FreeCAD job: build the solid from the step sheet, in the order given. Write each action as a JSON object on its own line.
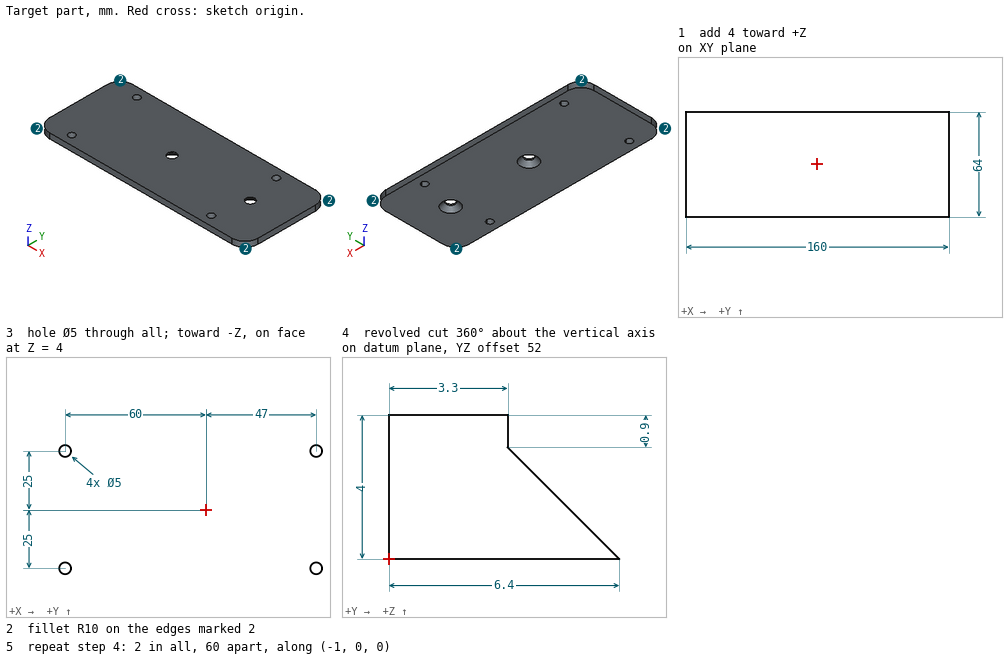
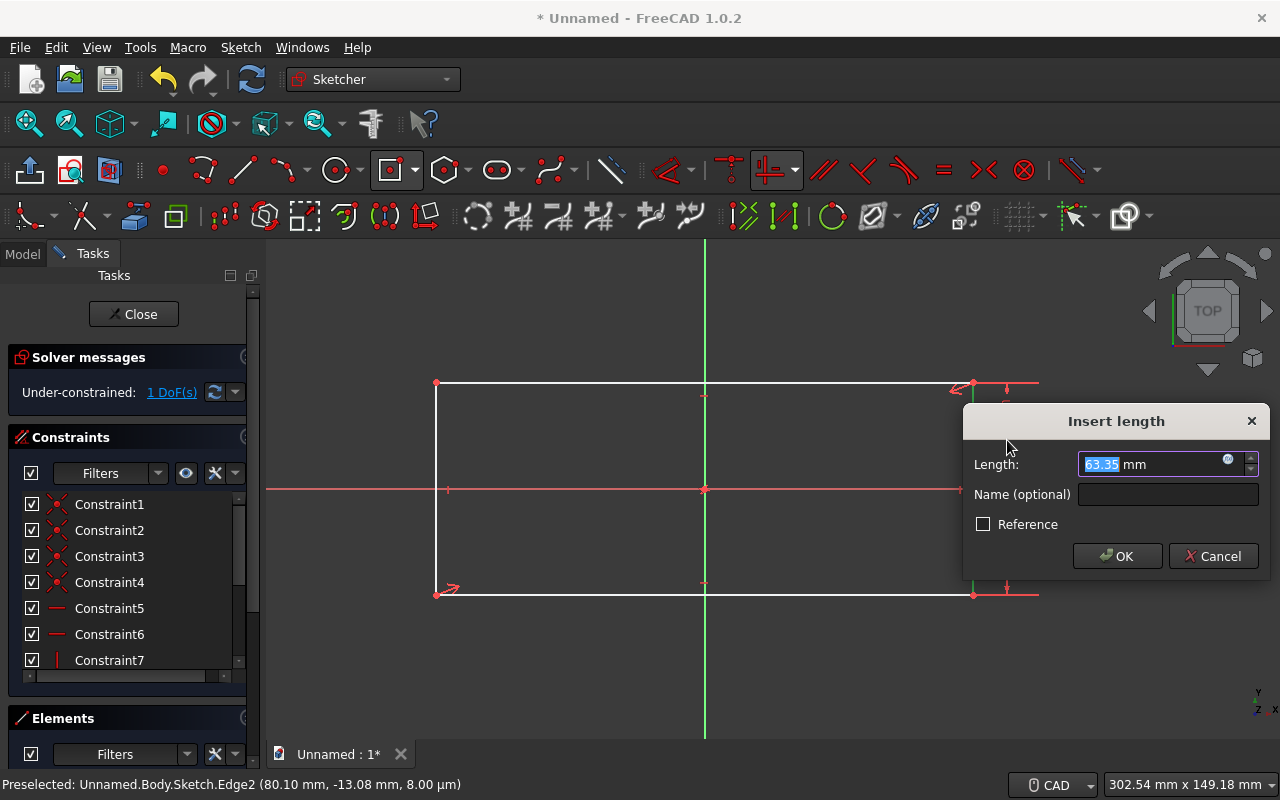
{"action": "type", "text": "64"}
{"action": "key", "text": "Return"}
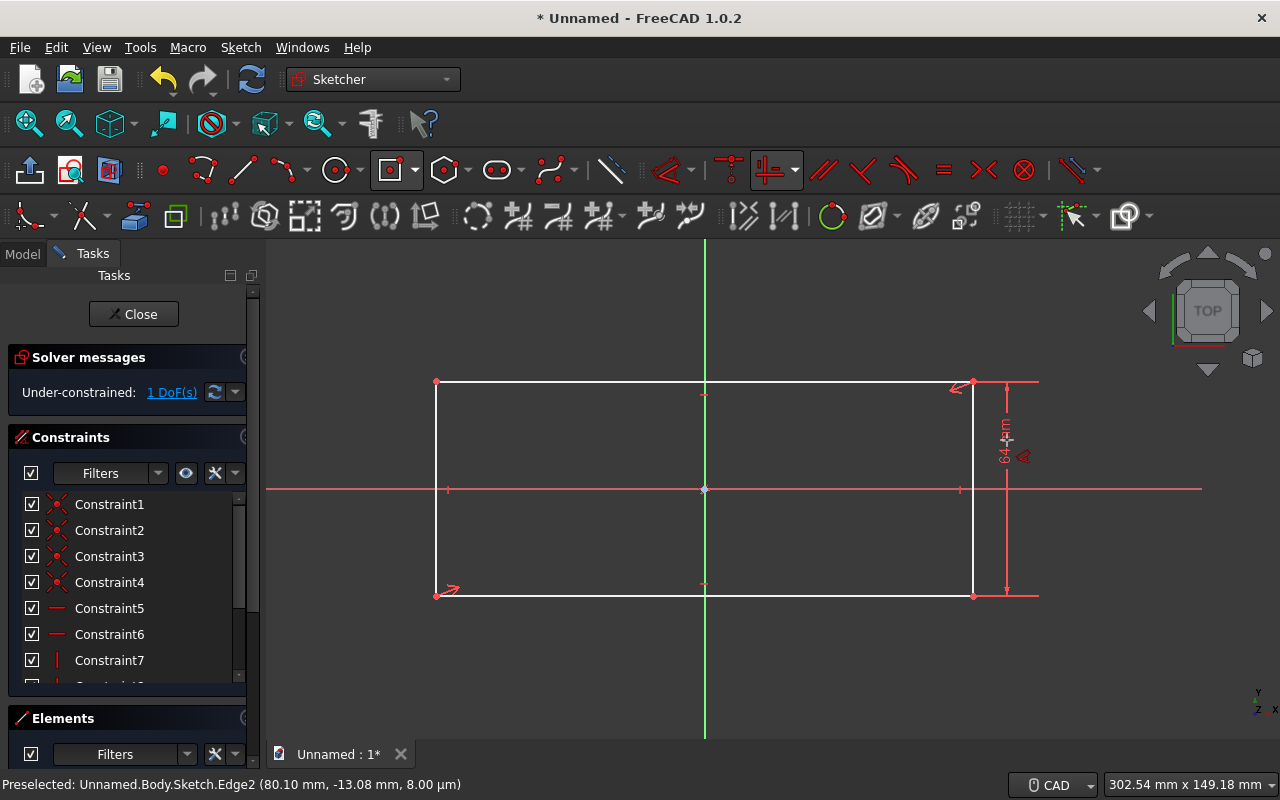
{"action": "left_click", "coordinate": [597, 596]}
{"action": "left_click", "coordinate": [581, 630]}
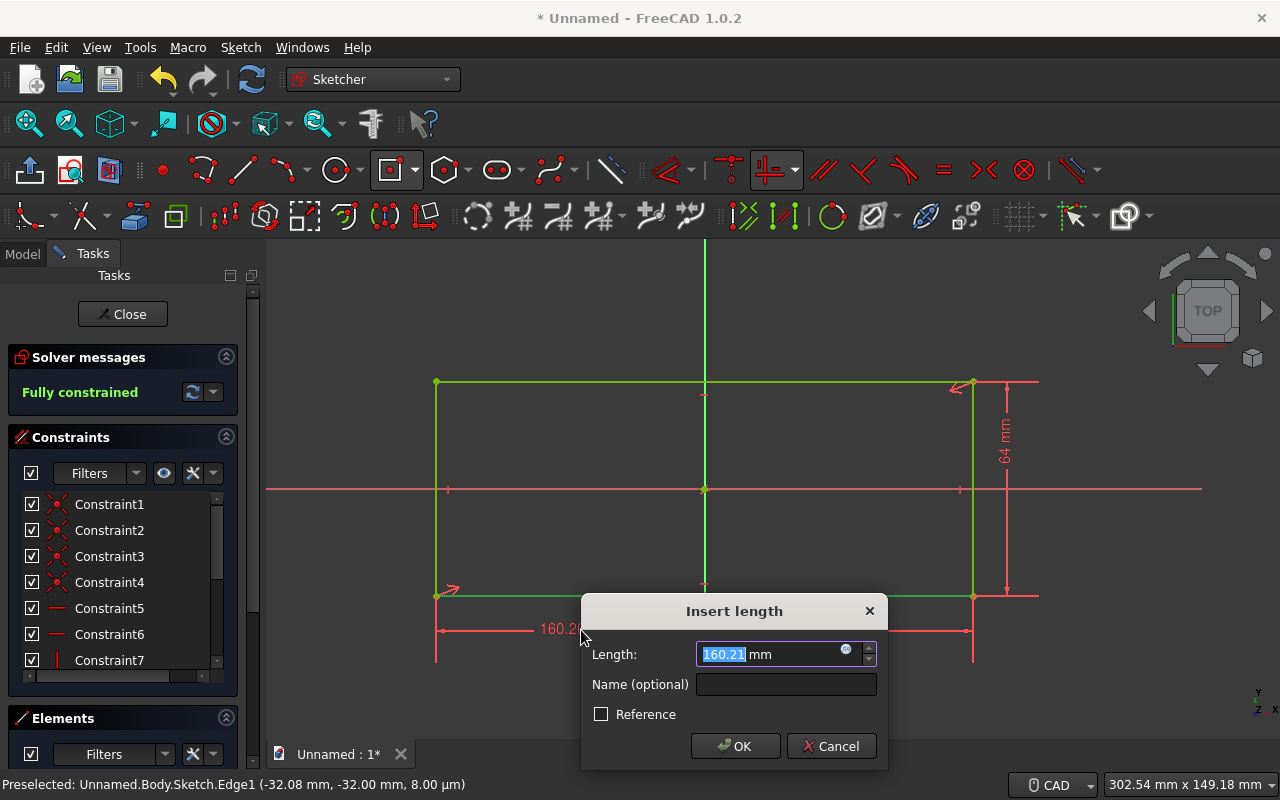
{"action": "type", "text": "160"}
{"action": "key", "text": "Return"}
{"action": "key", "text": "Escape"}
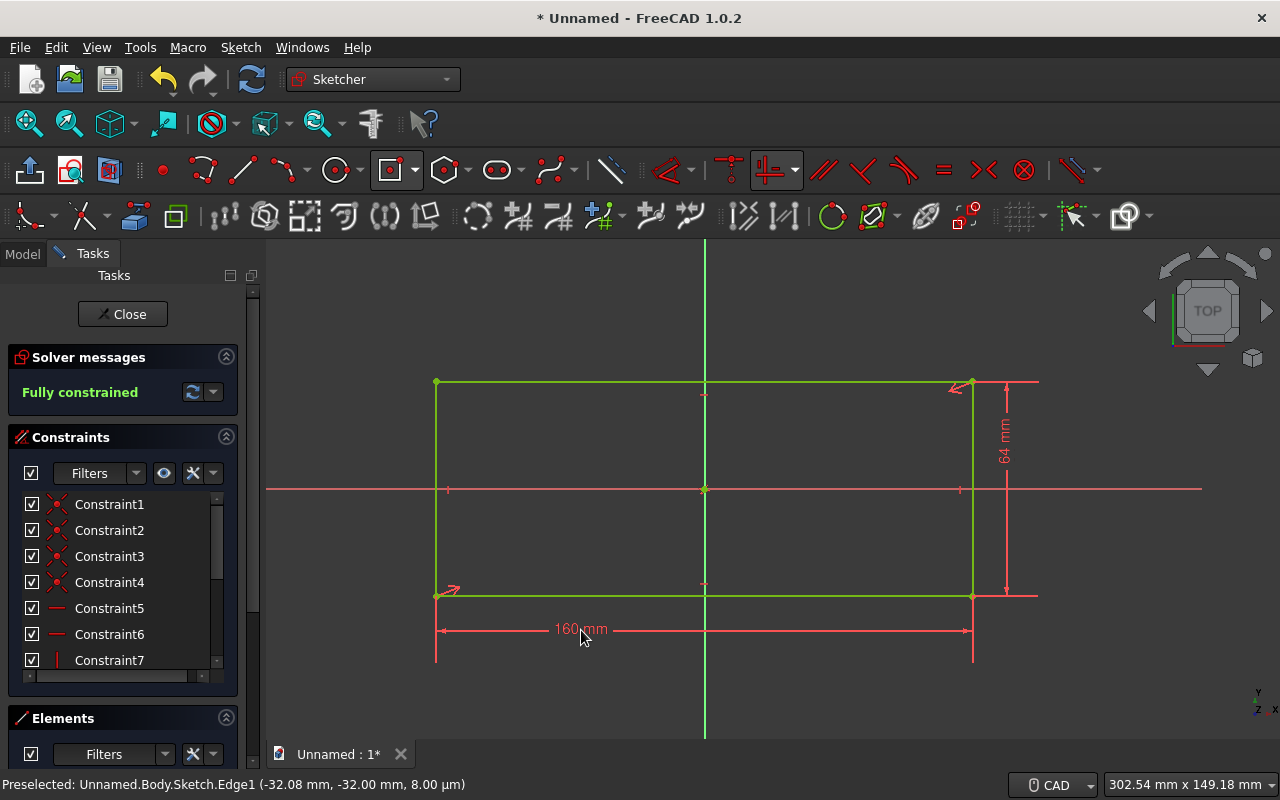
{"action": "left_click", "coordinate": [123, 314]}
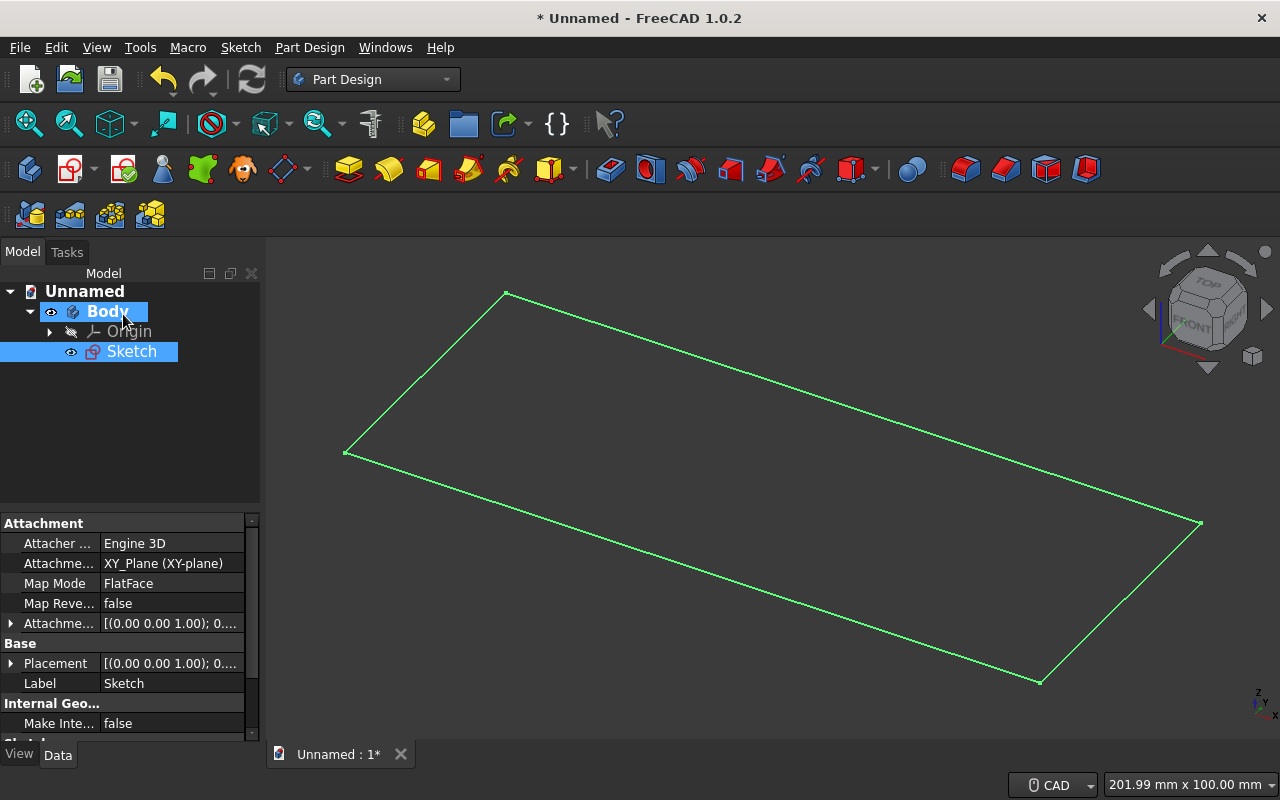
{"action": "left_click", "coordinate": [350, 170]}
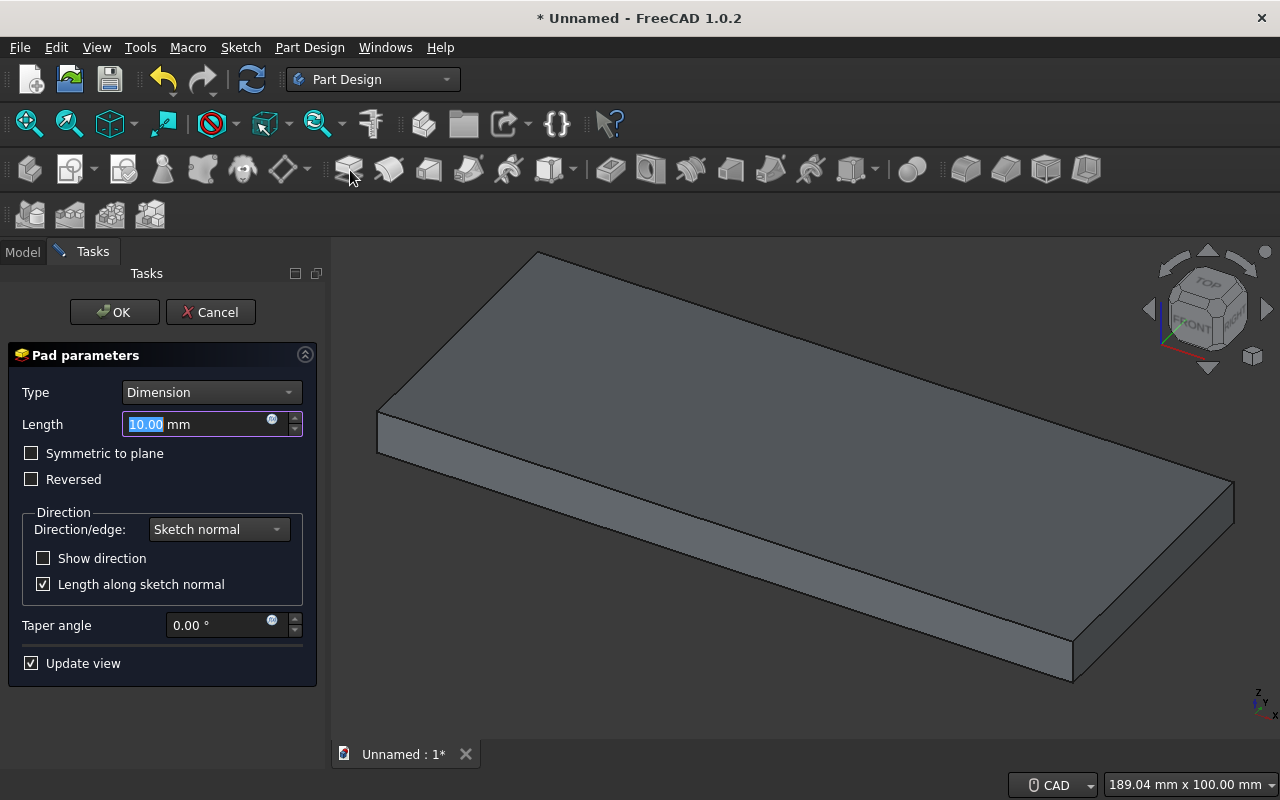
{"action": "type", "text": "4"}
{"action": "key", "text": "Tab"}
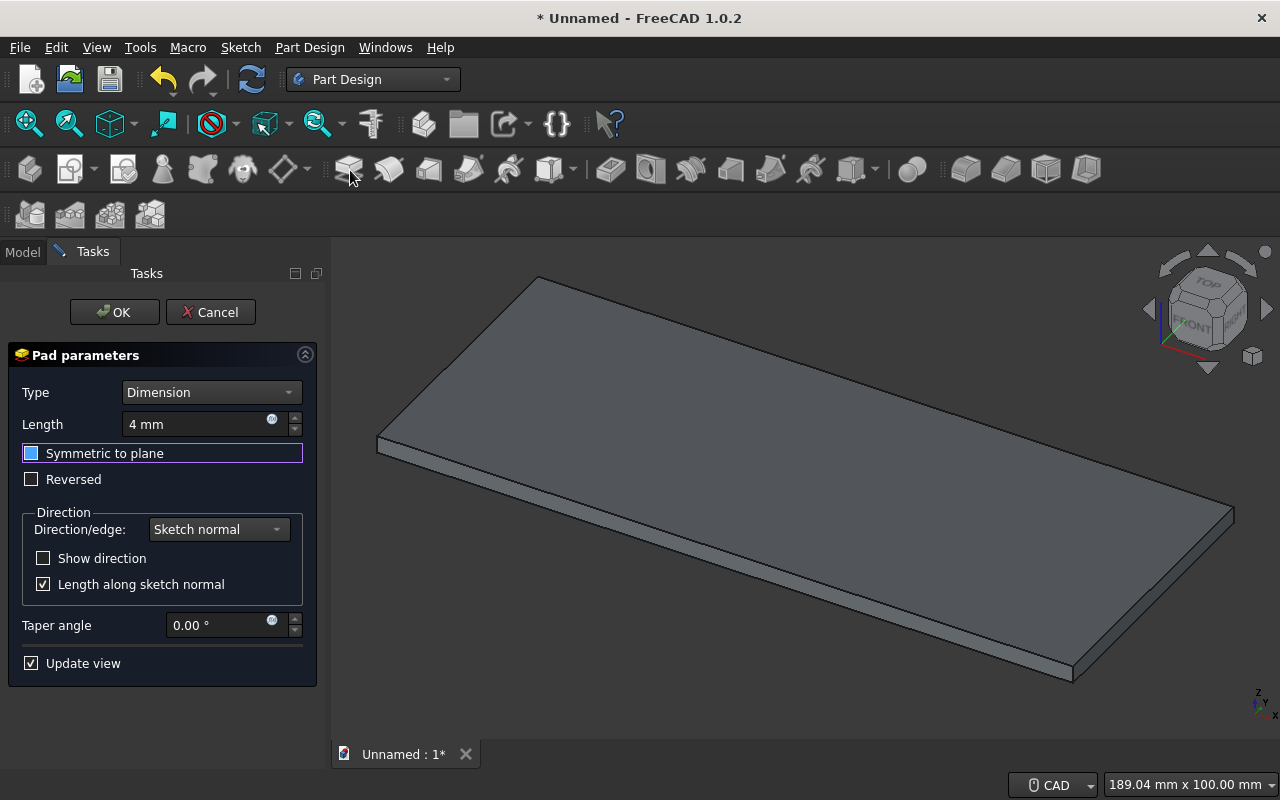
{"action": "left_click", "coordinate": [115, 312]}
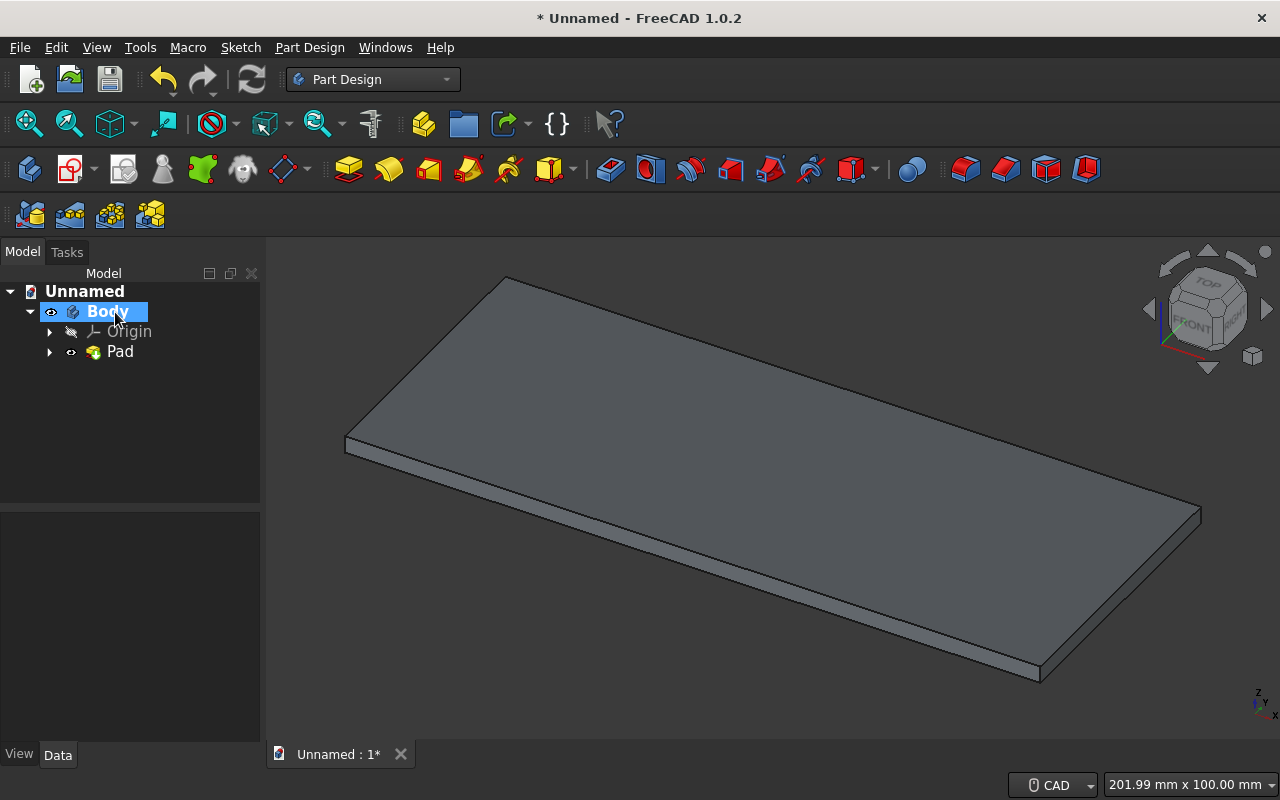
{"action": "left_click", "coordinate": [1040, 674]}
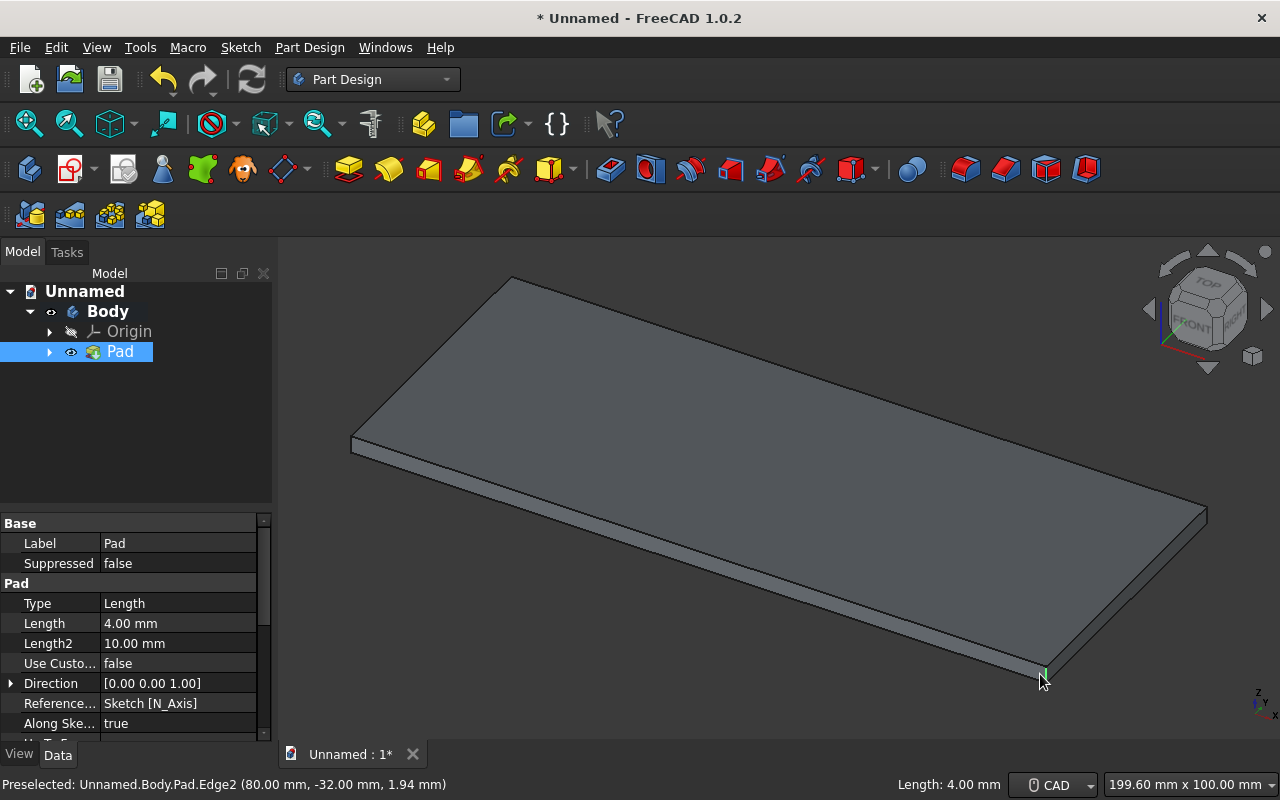
{"action": "scroll", "coordinate": [351, 443], "scroll_direction": "up", "scroll_amount": 4}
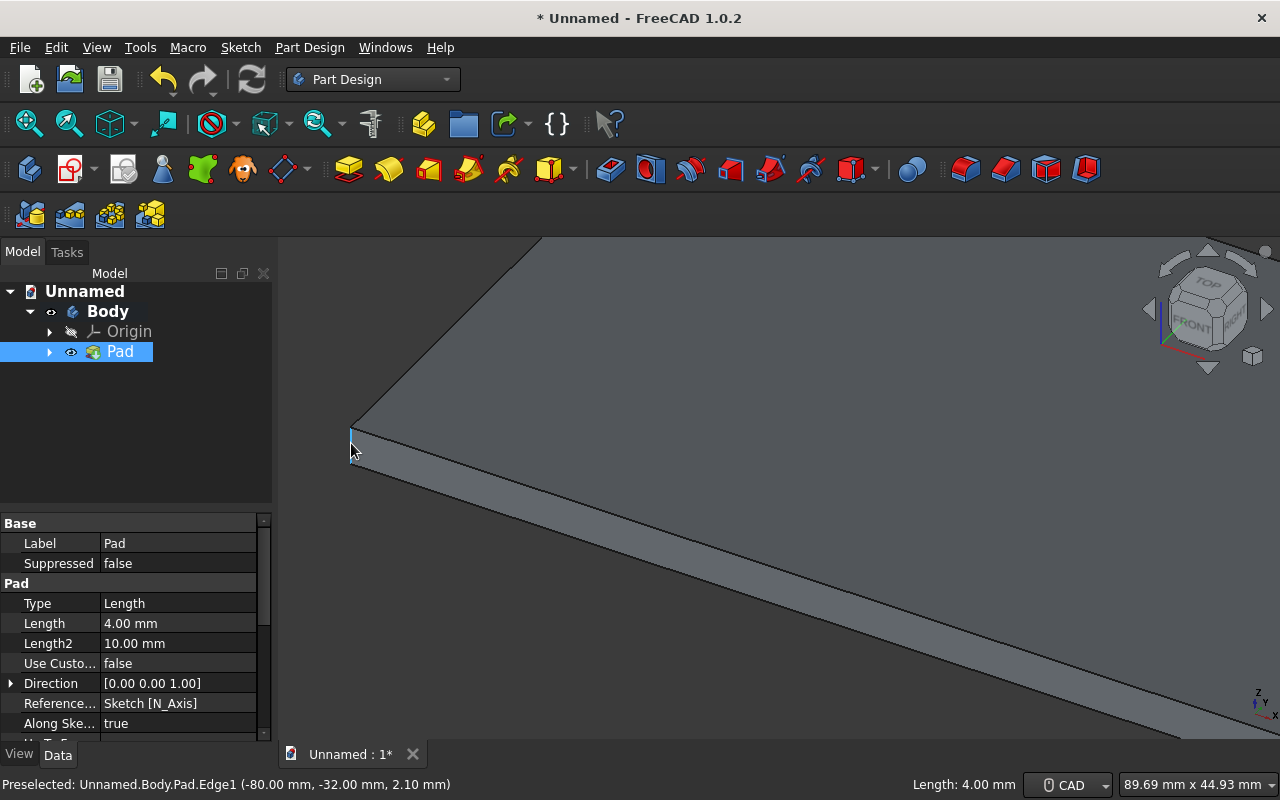
{"action": "left_click", "coordinate": [30, 124]}